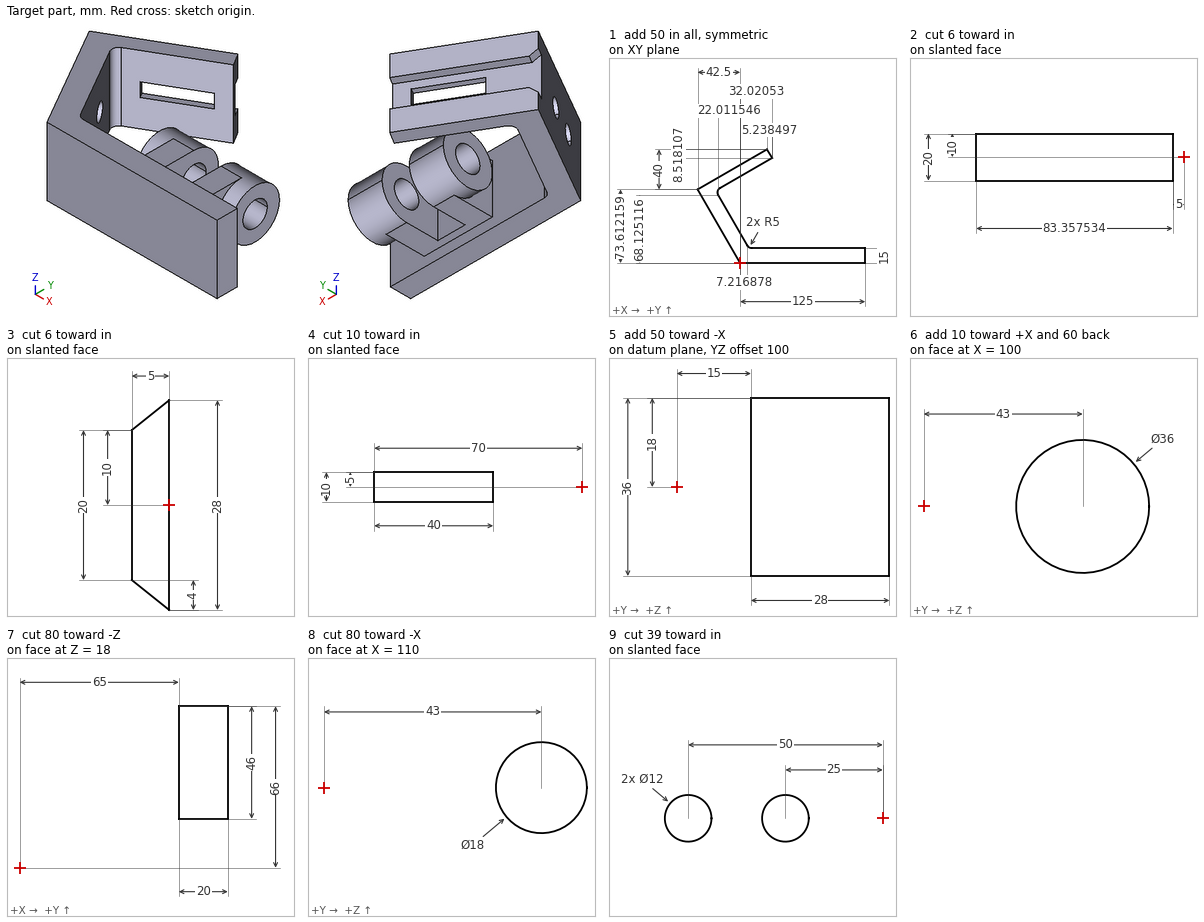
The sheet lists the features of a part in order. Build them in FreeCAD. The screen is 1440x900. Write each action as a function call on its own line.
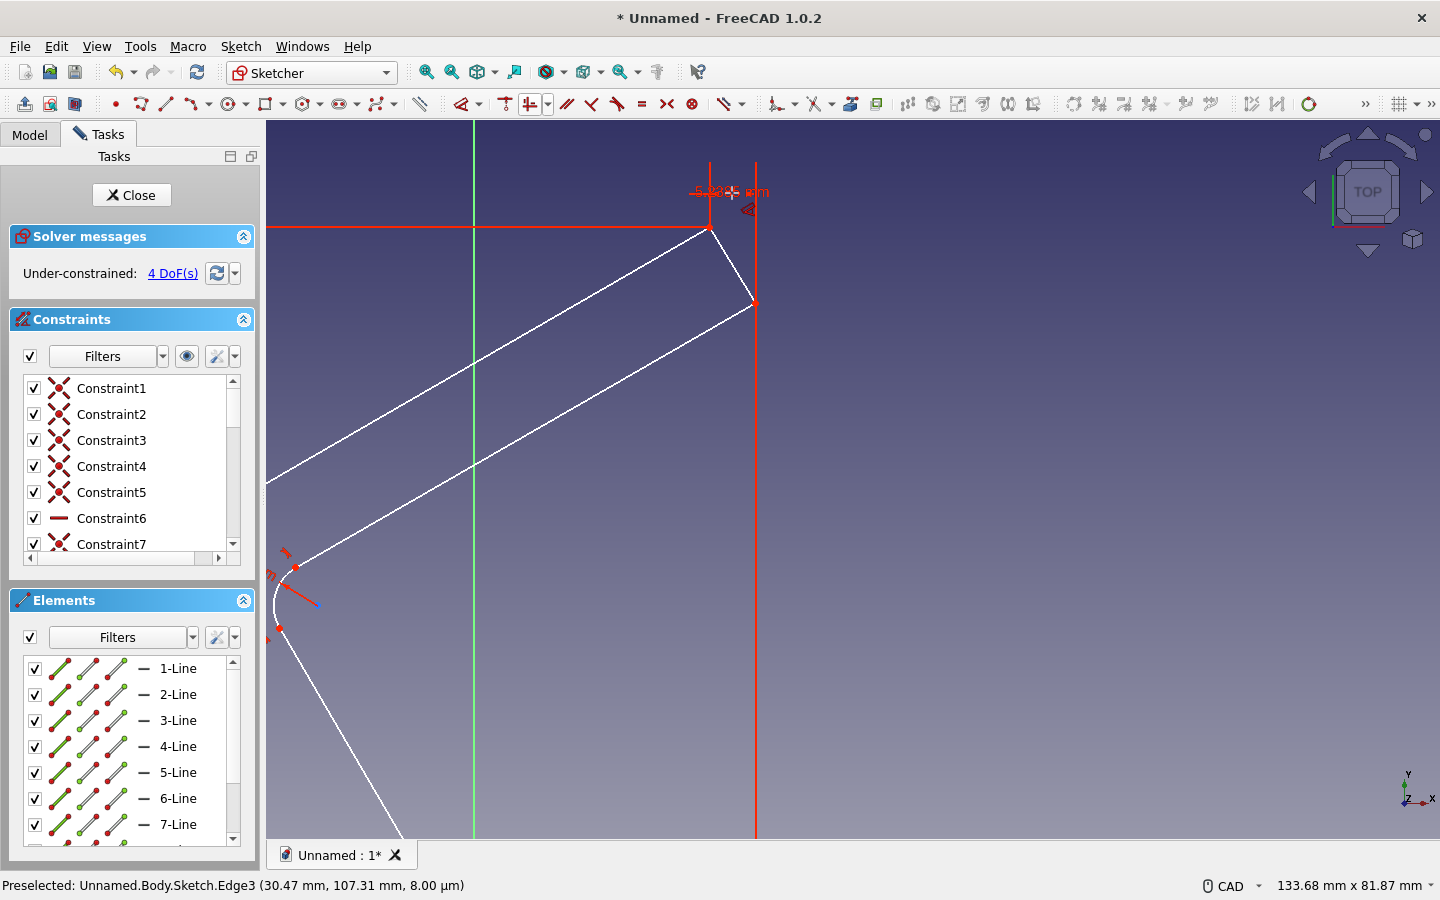
click(742, 280)
click(676, 265)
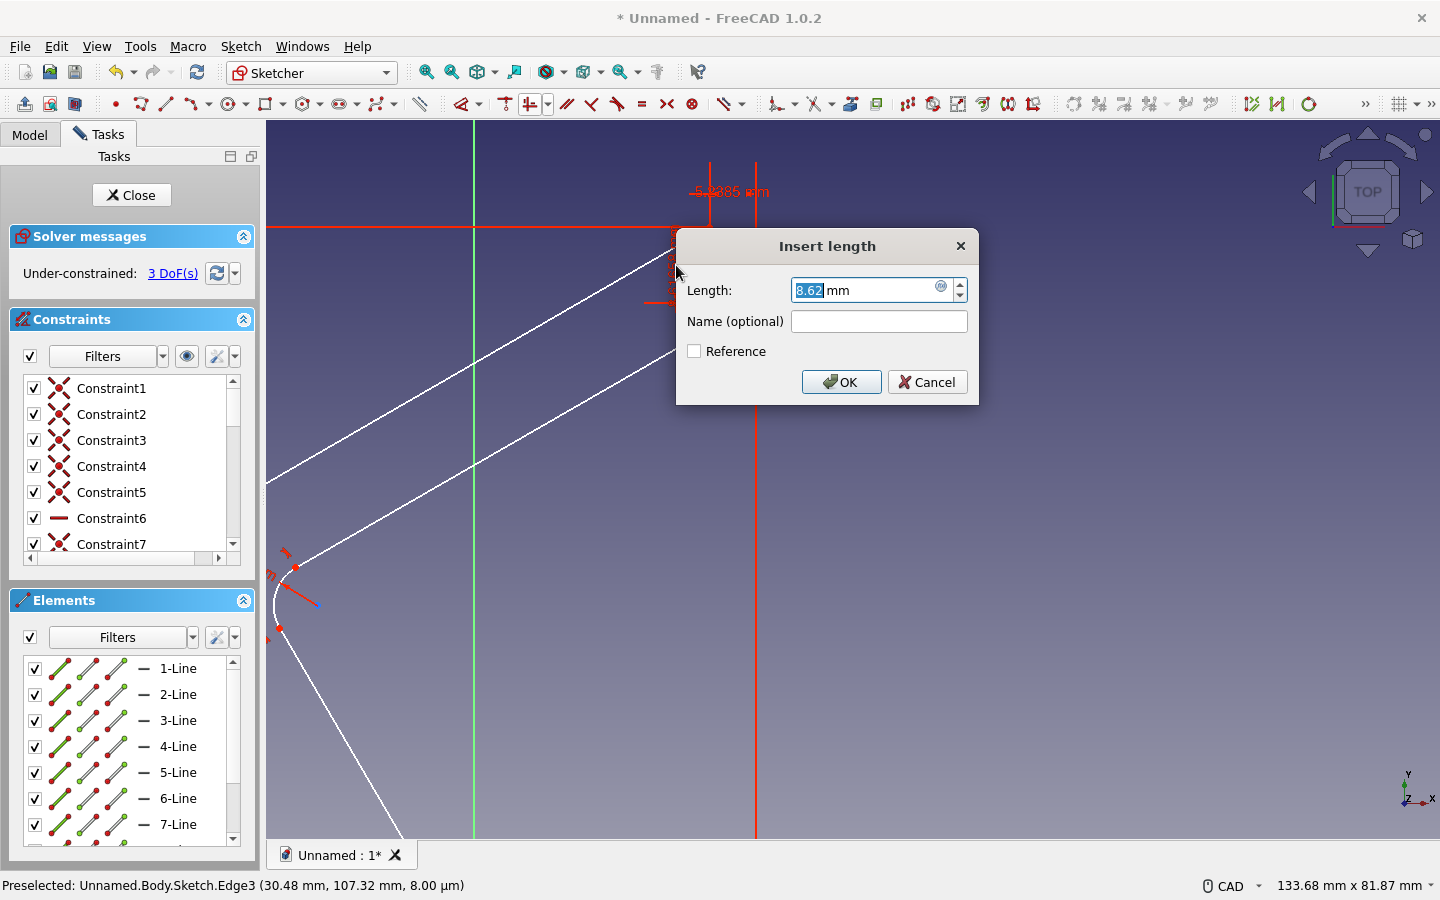
text(8.518107)
key(Return)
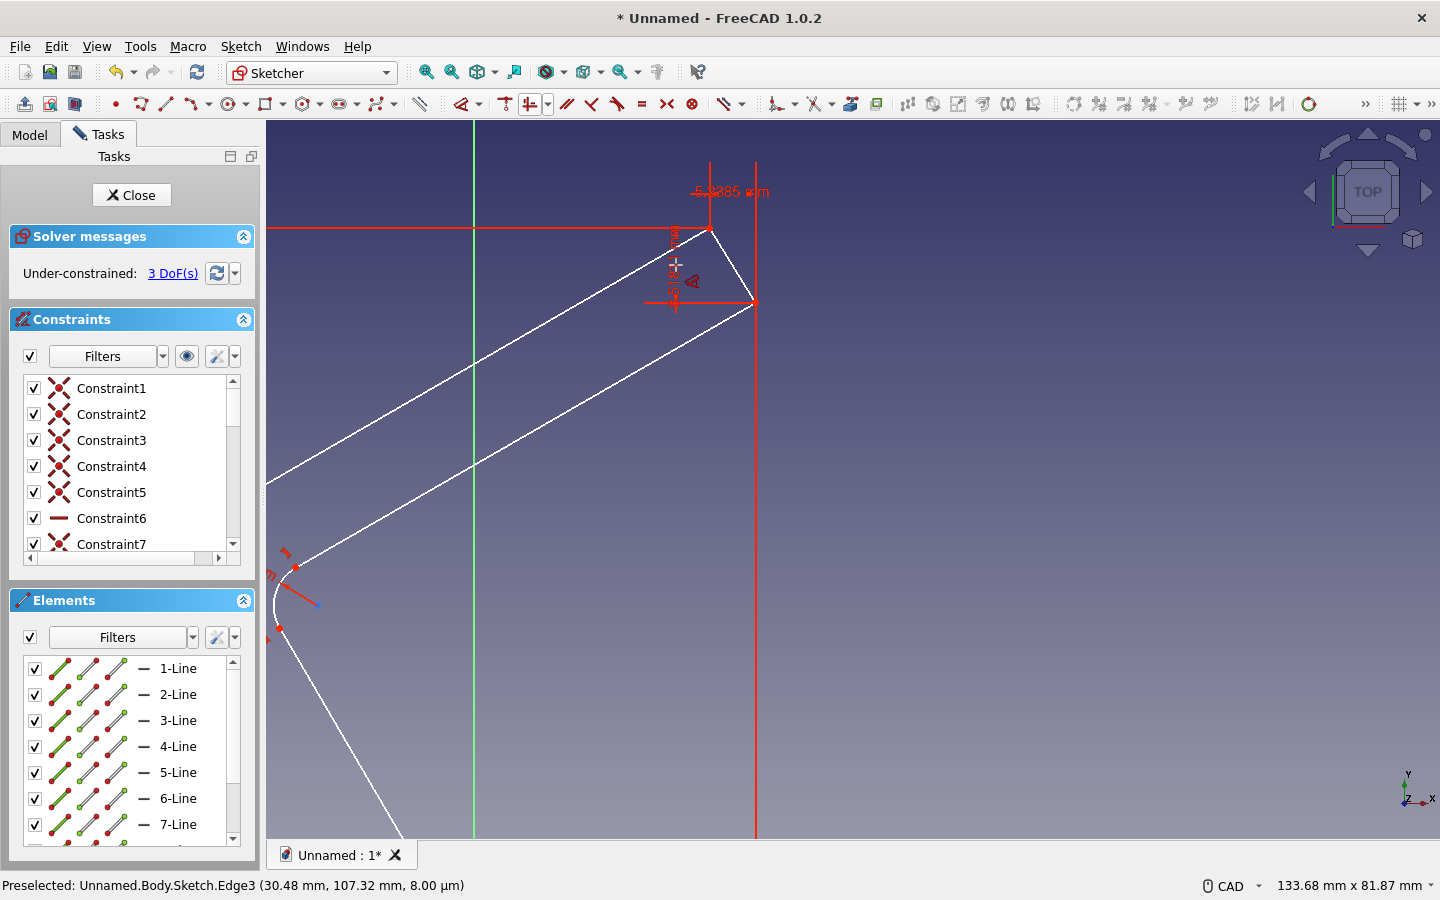
scroll(742, 280, down, 4)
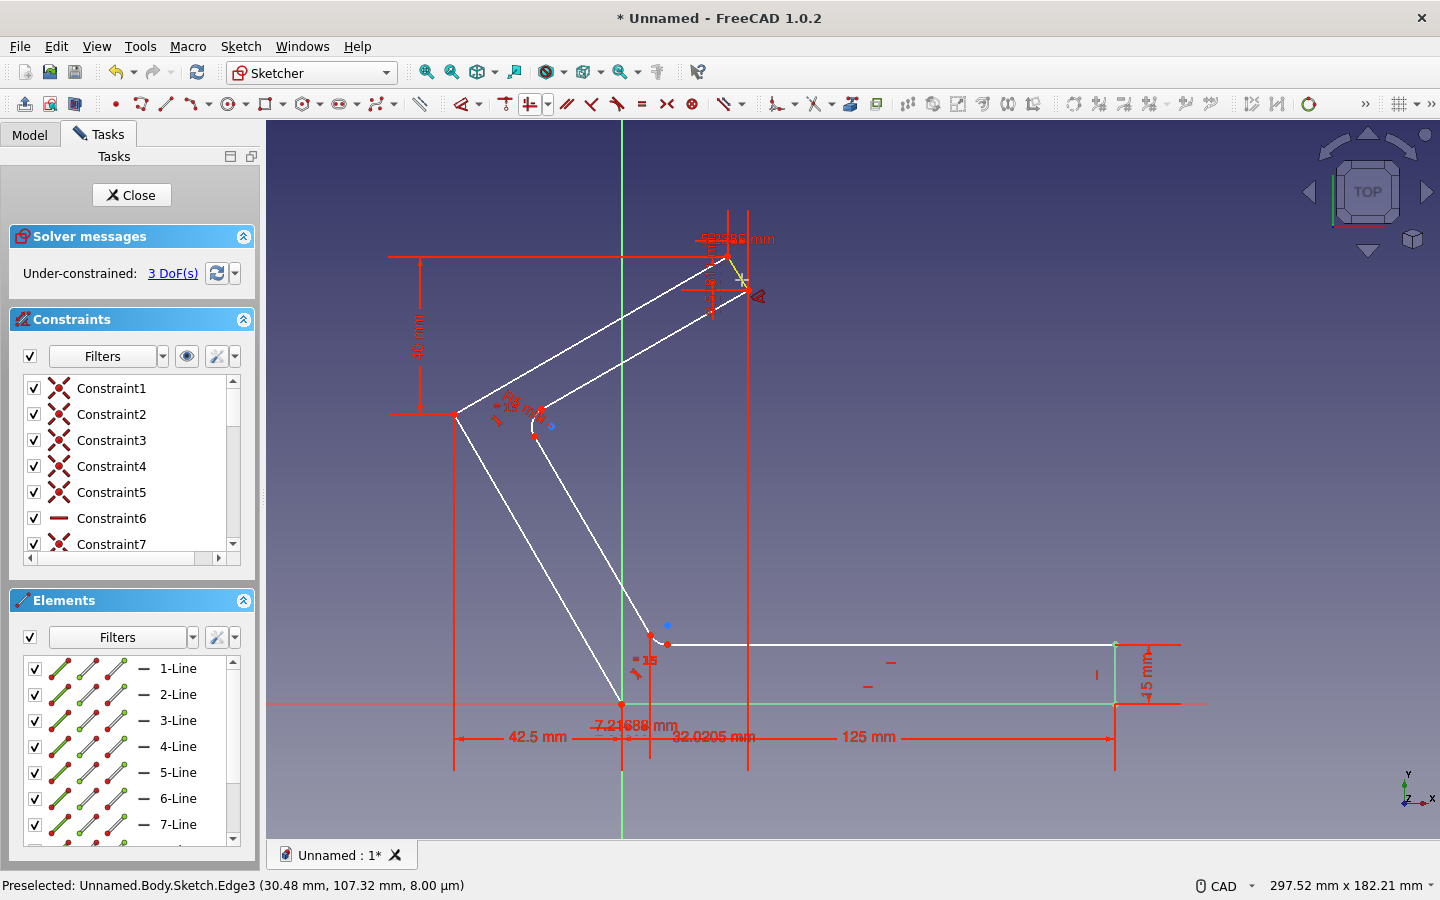
click(535, 437)
click(598, 403)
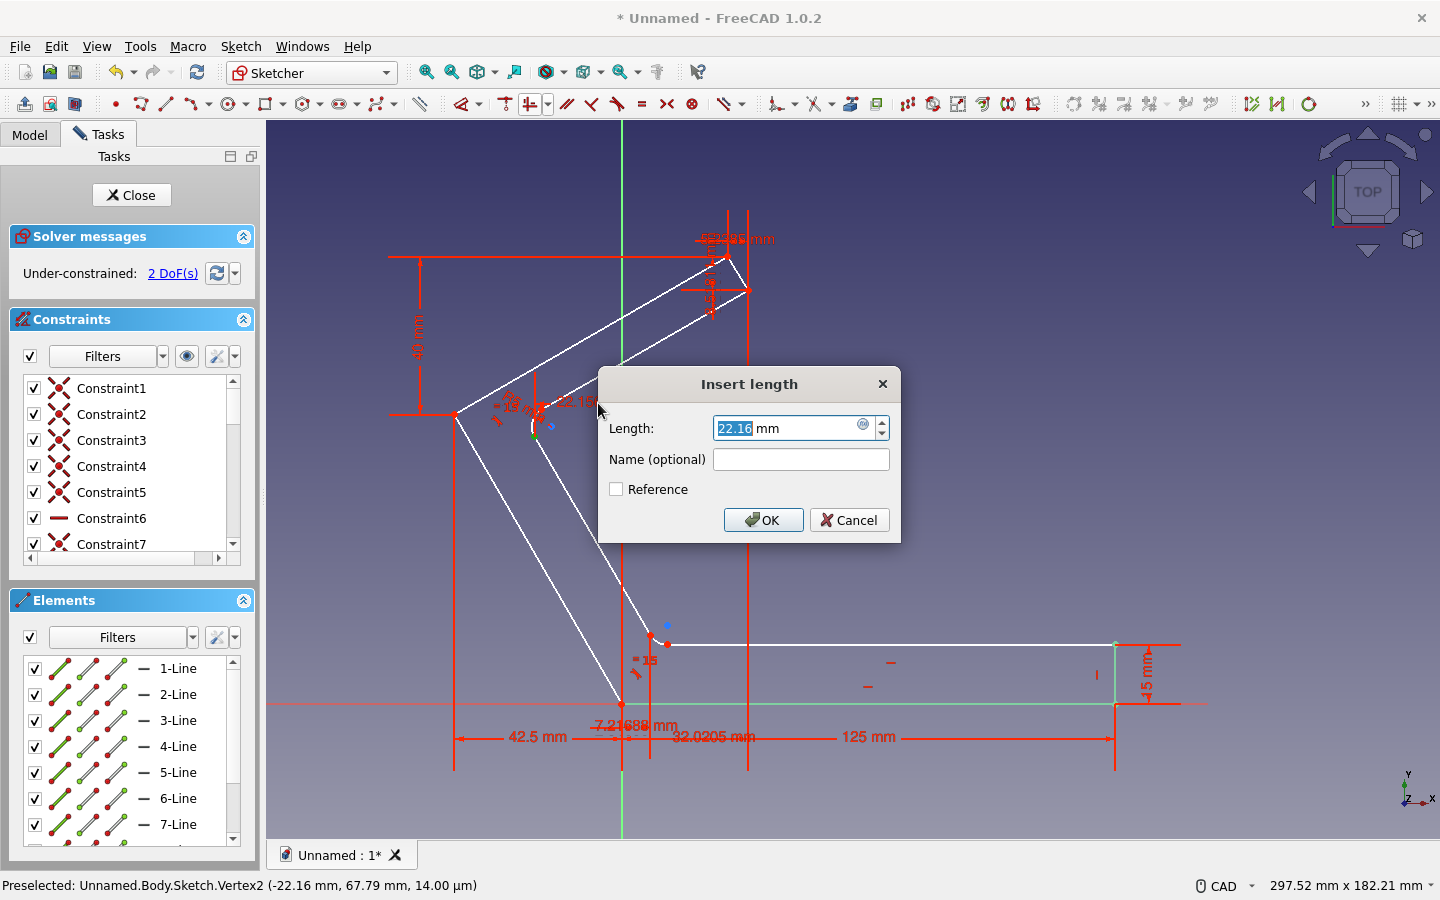
text(22.011546)
key(Return)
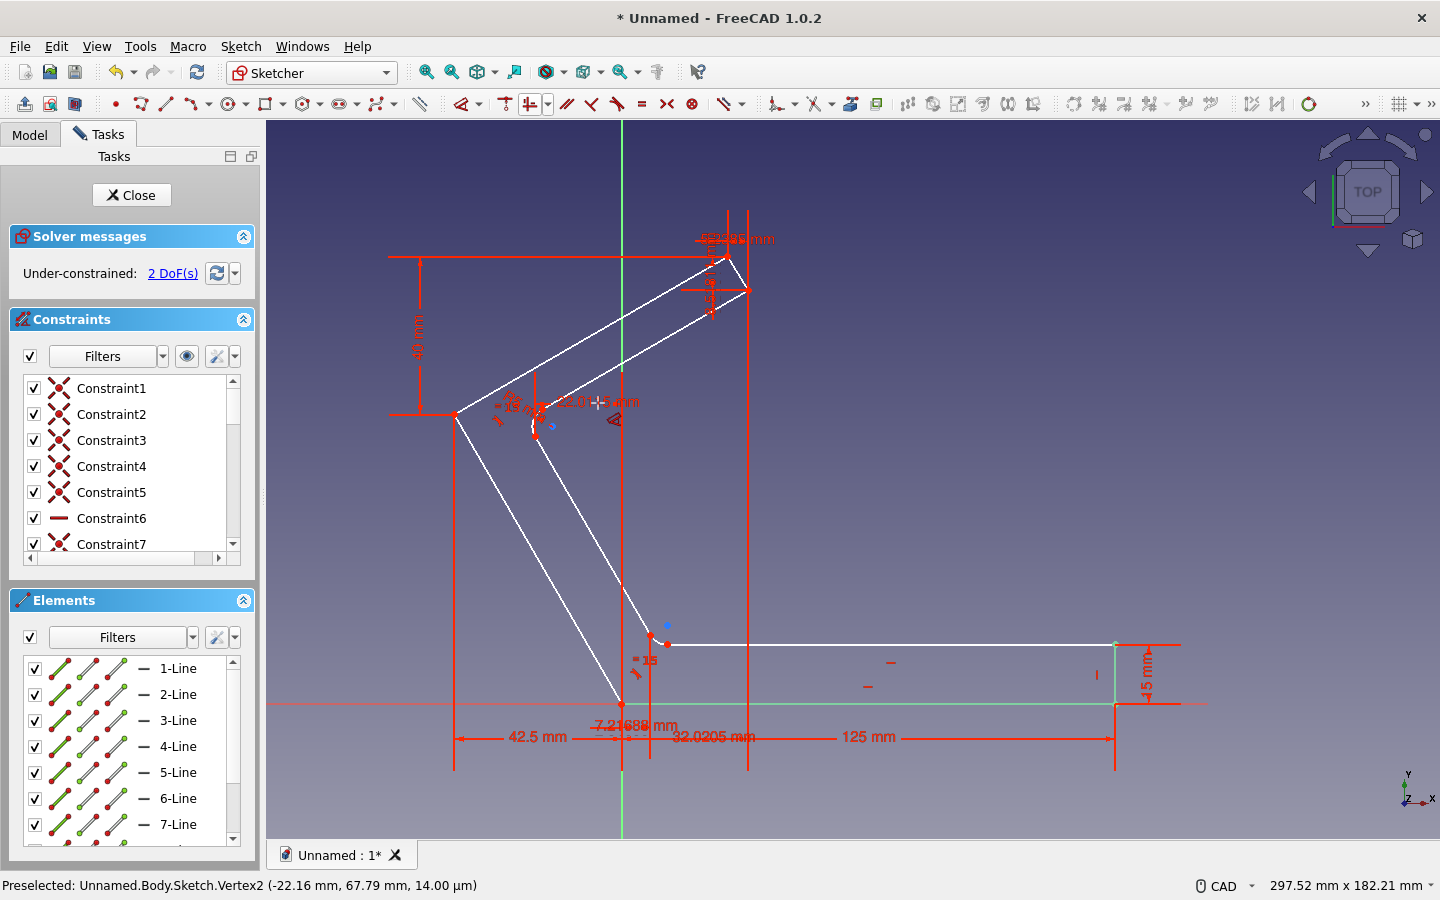
click(535, 437)
click(501, 570)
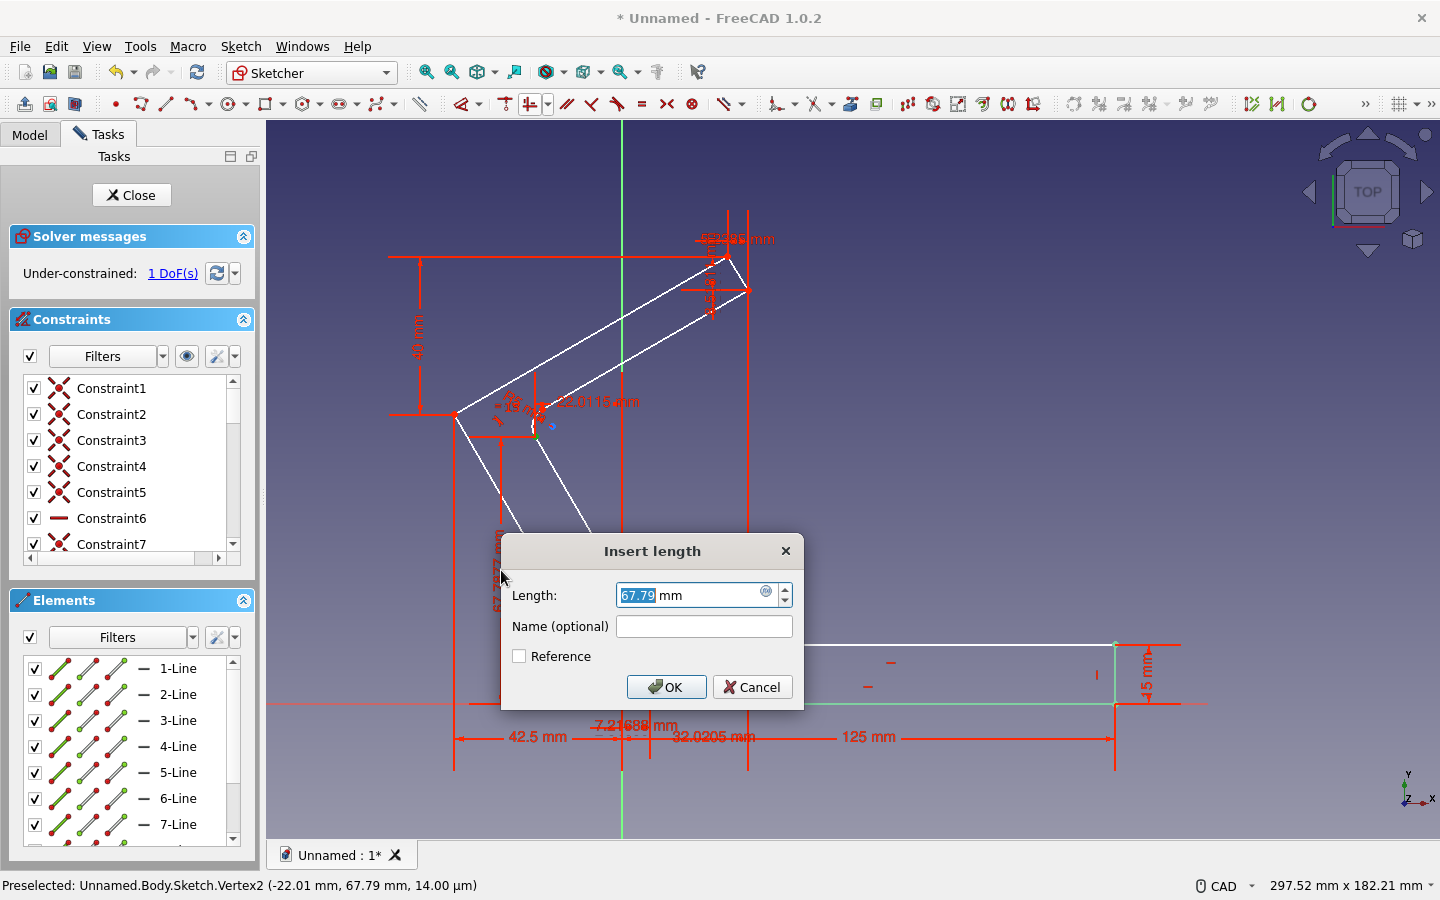
text(68.125116)
key(Return)